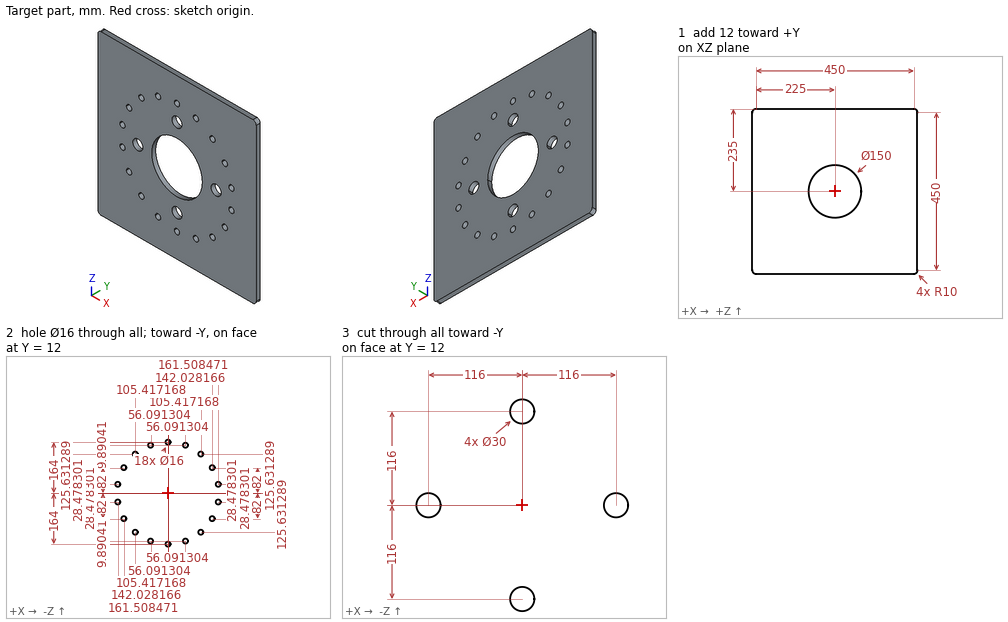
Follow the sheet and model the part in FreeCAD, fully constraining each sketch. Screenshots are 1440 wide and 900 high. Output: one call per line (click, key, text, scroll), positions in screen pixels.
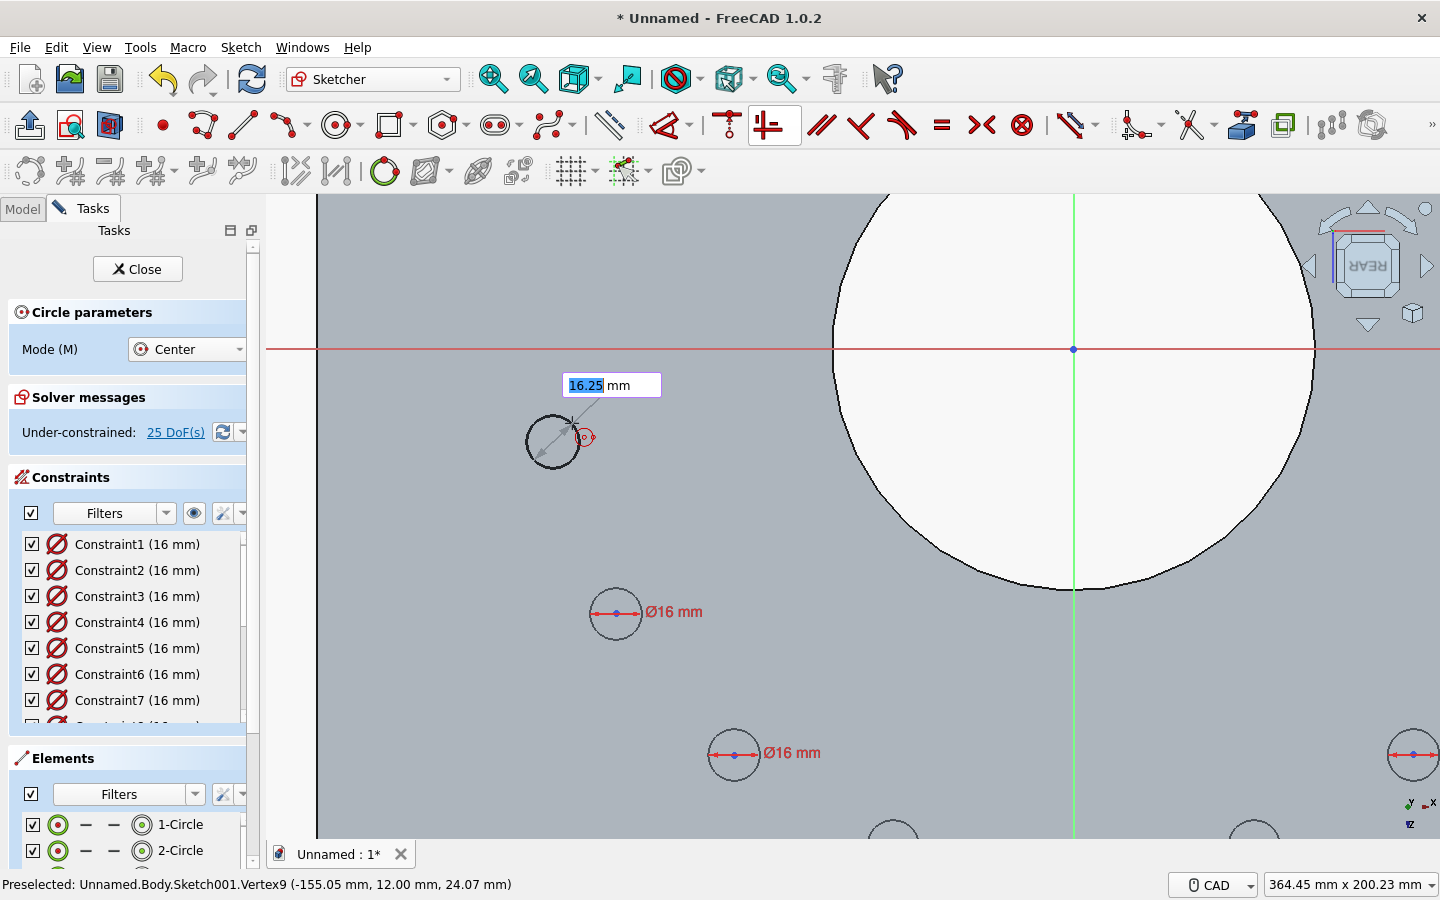
text(16)
key(Return)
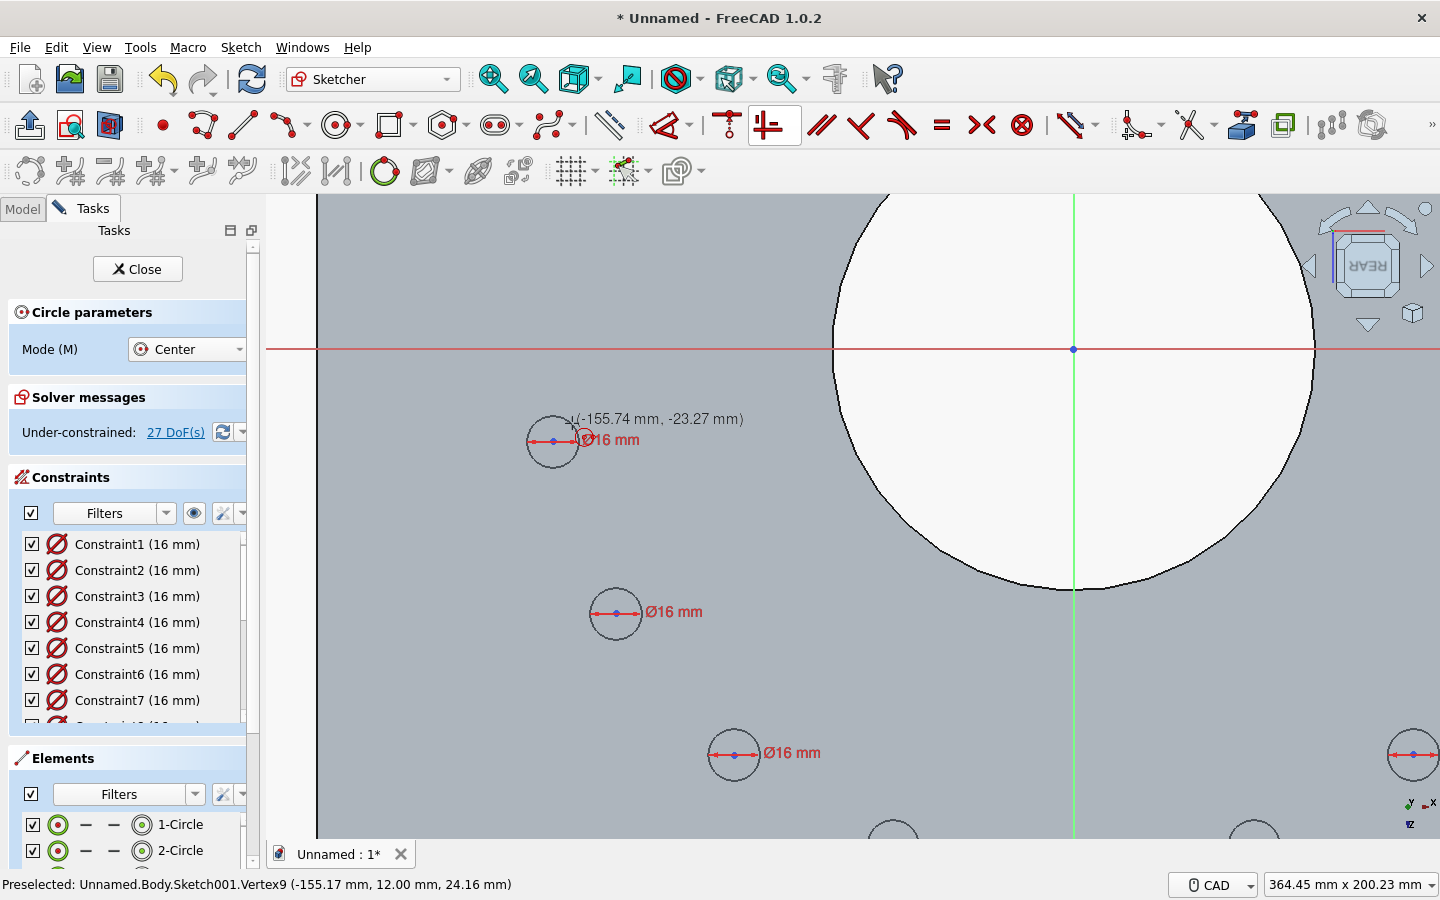
click(553, 257)
move(572, 239)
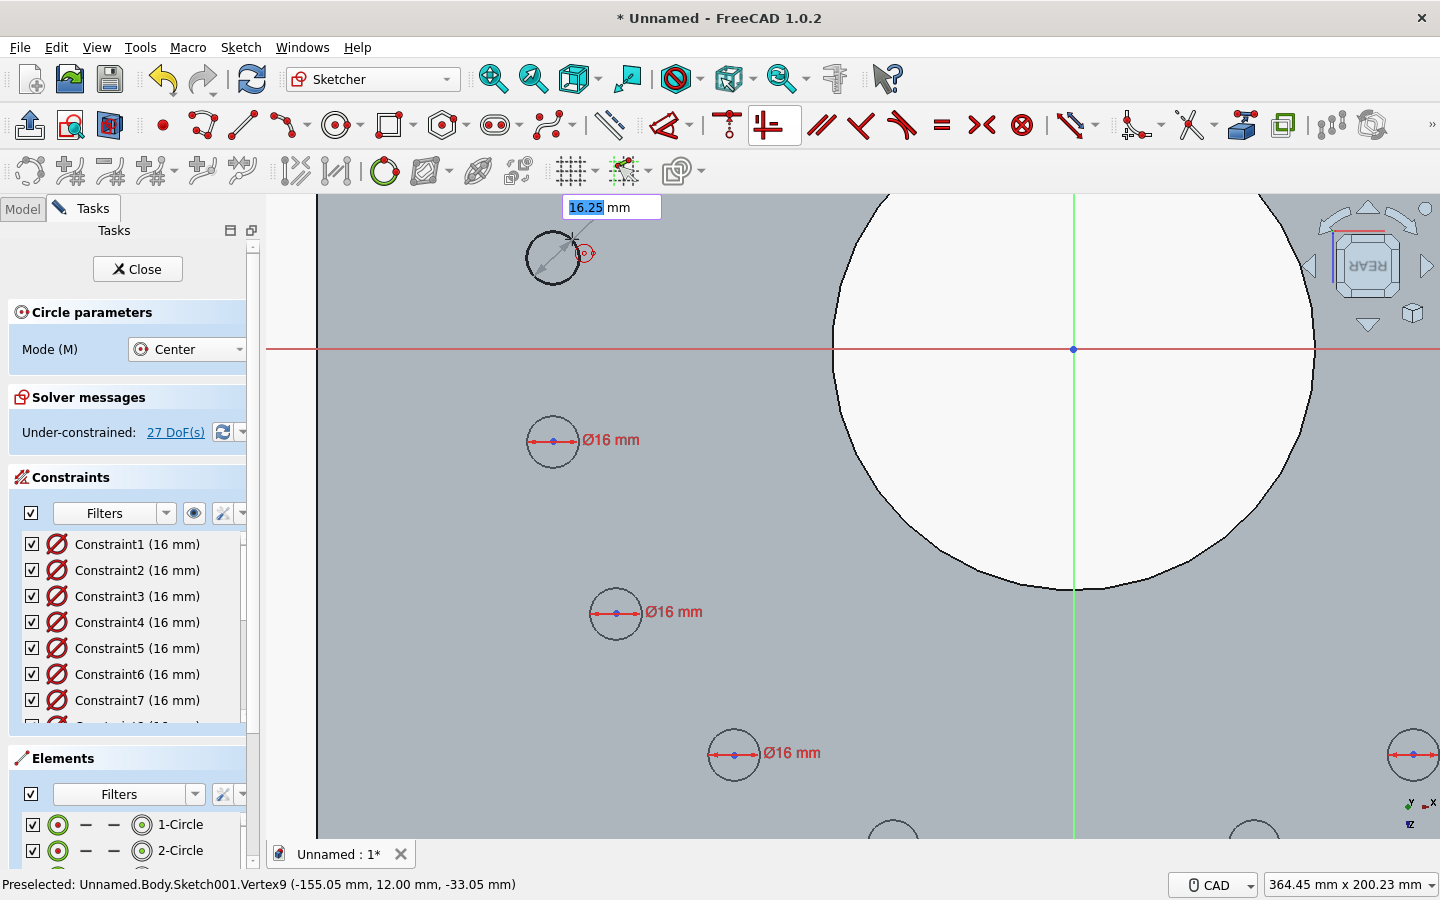
text(16)
key(Return)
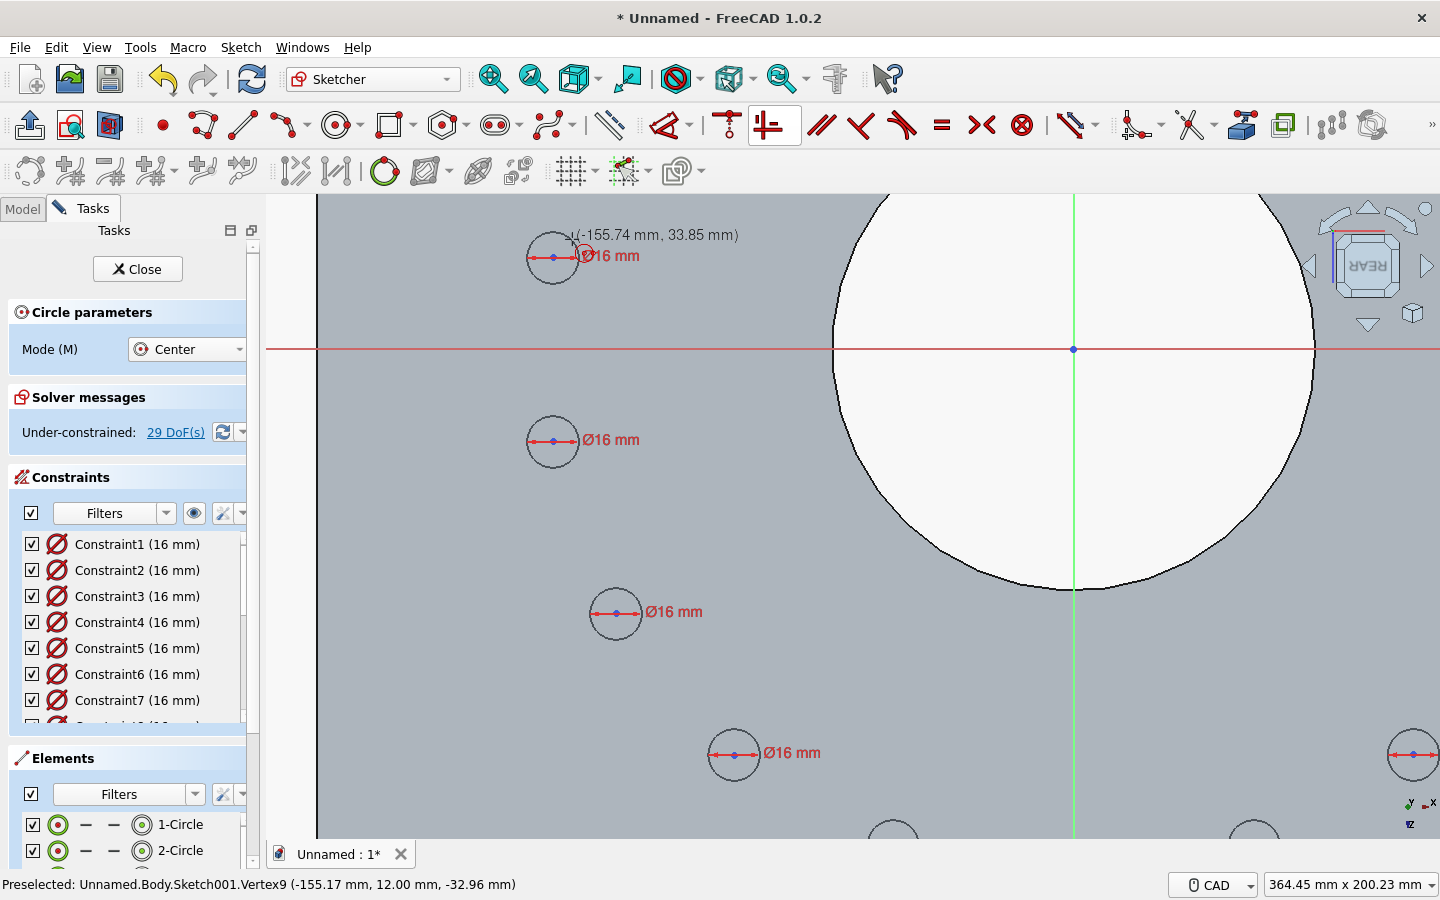
scroll(616, 614, down, 5)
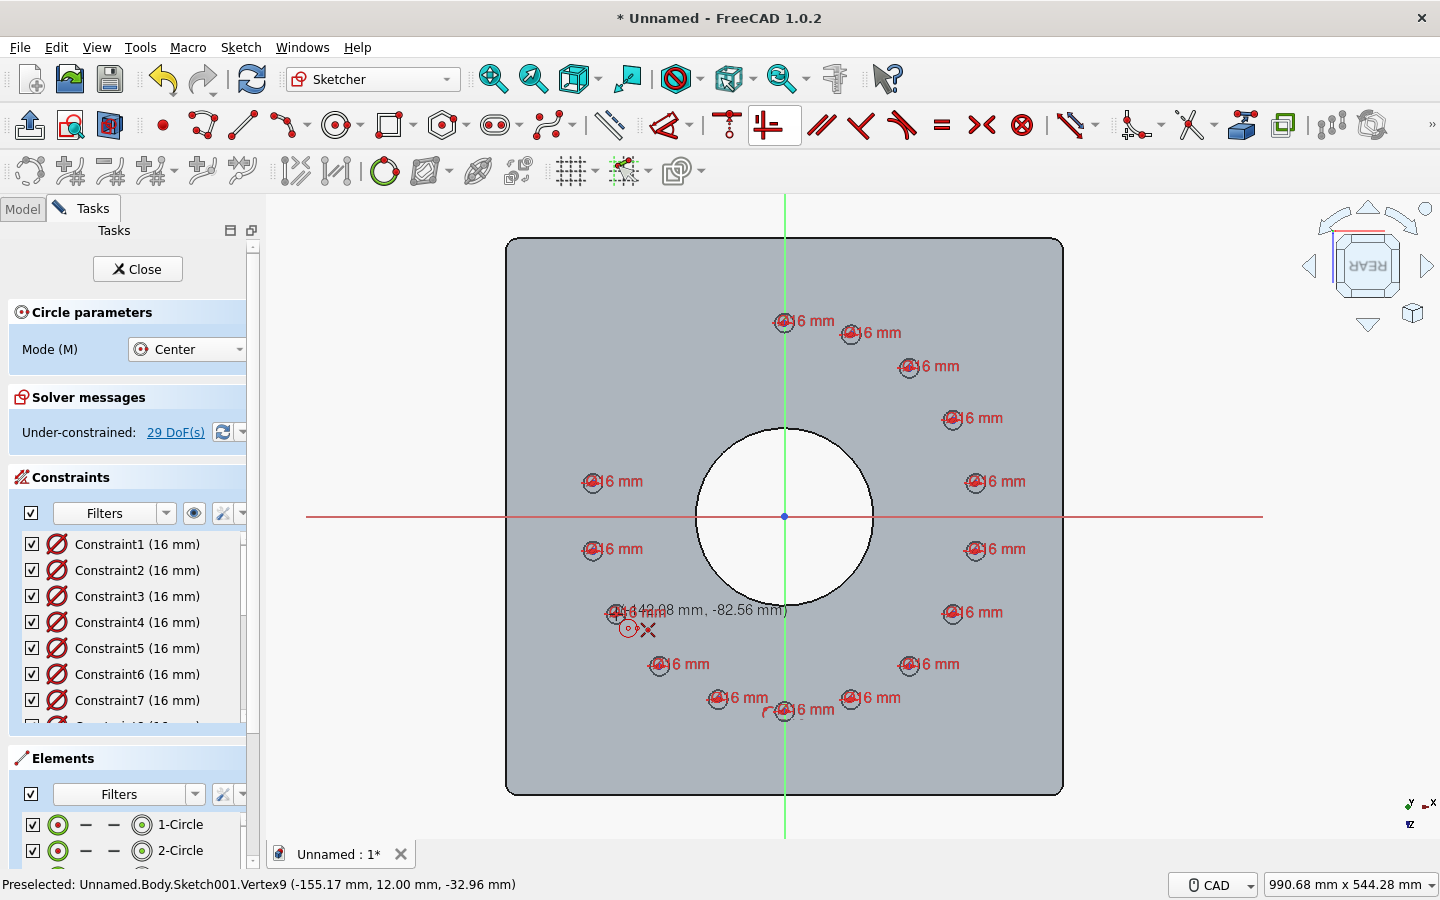
scroll(616, 420, up, 5)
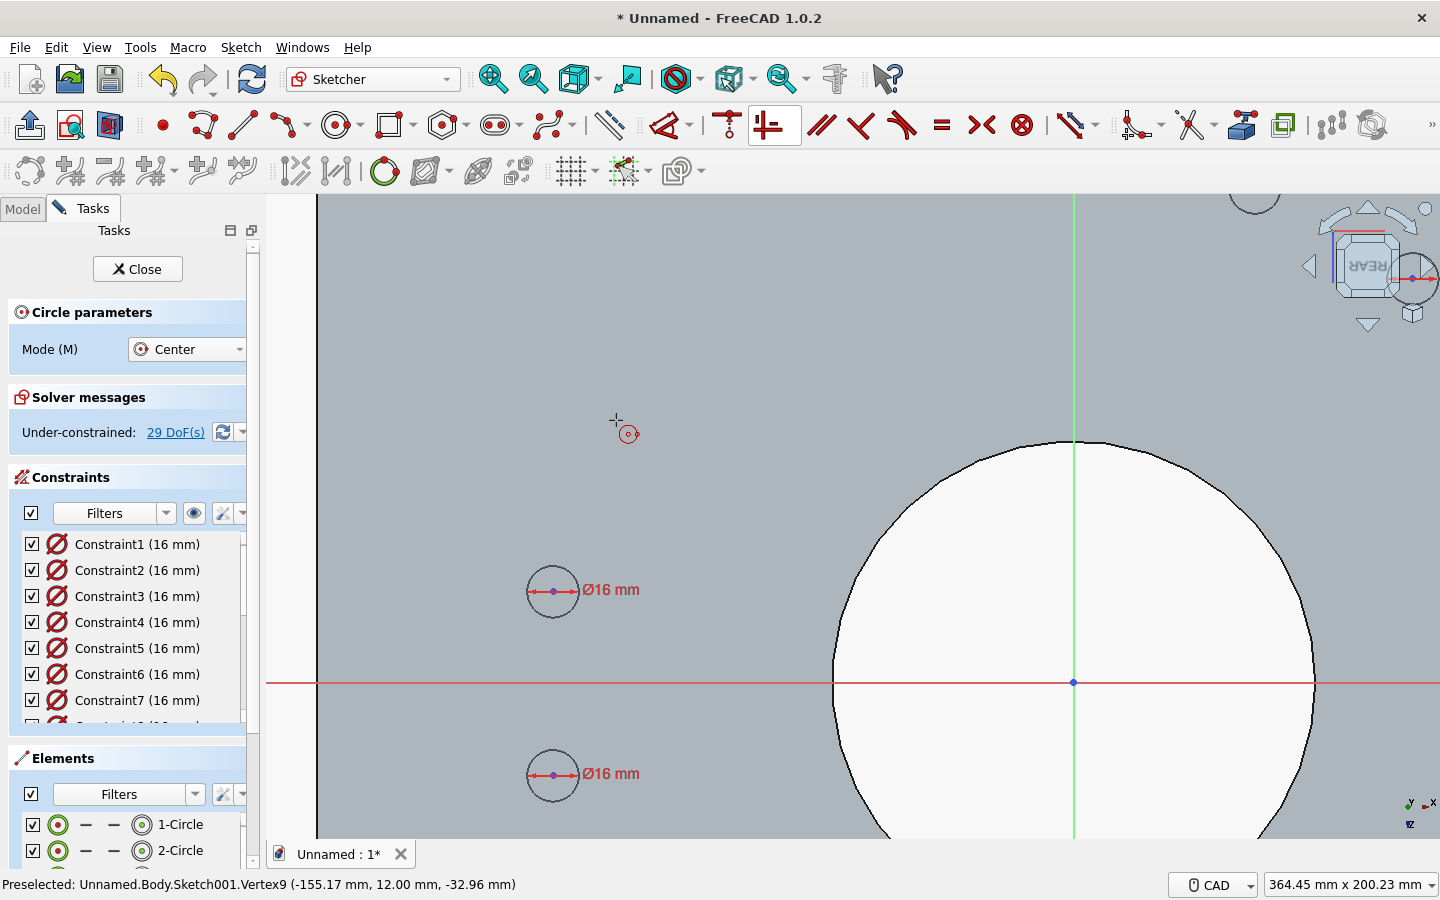
click(616, 419)
move(634, 401)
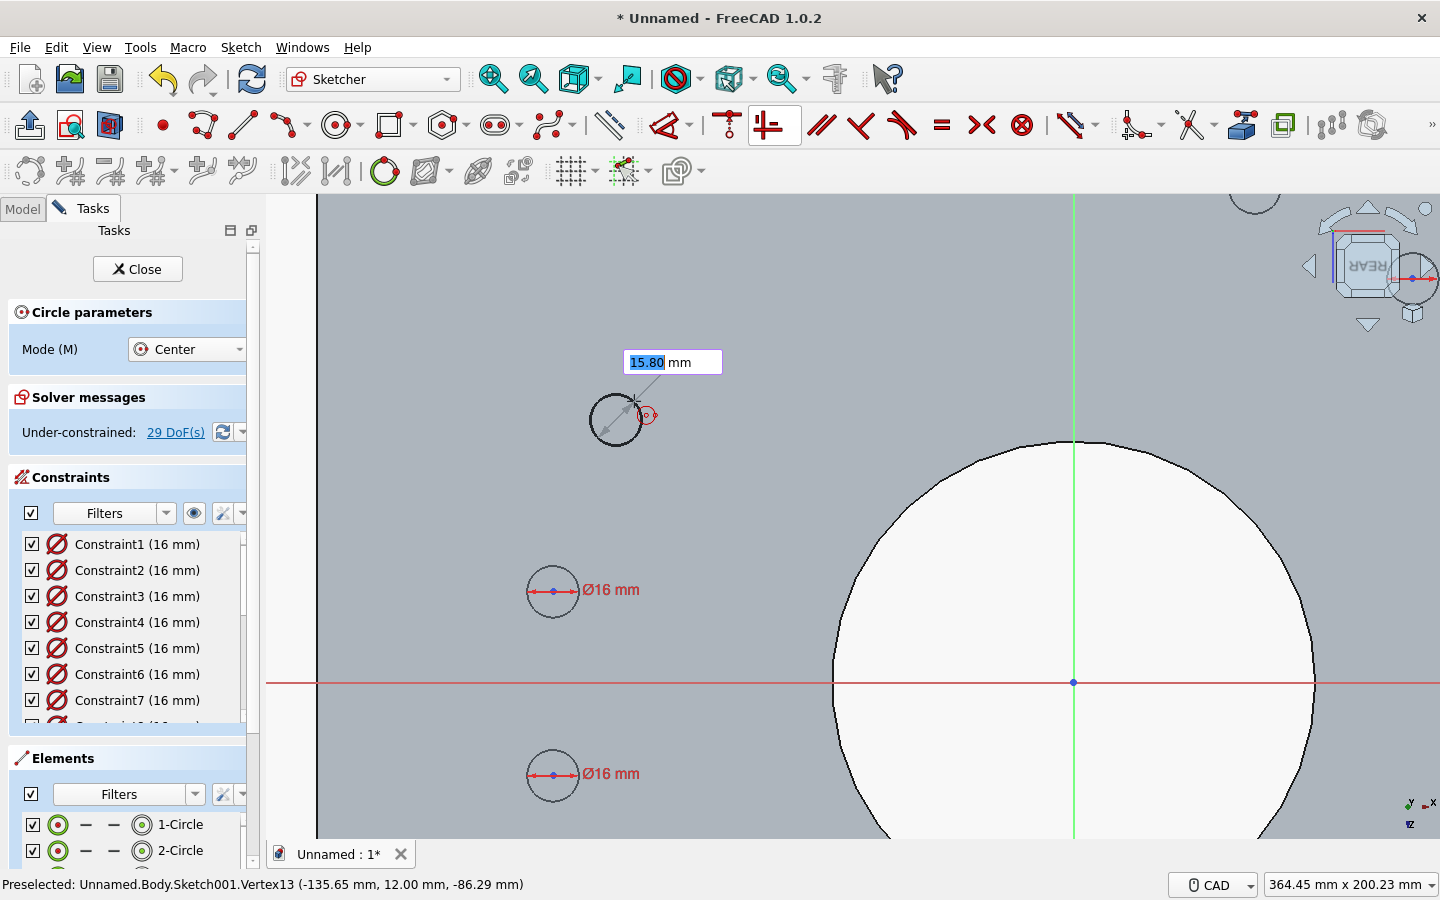
text(16)
key(Return)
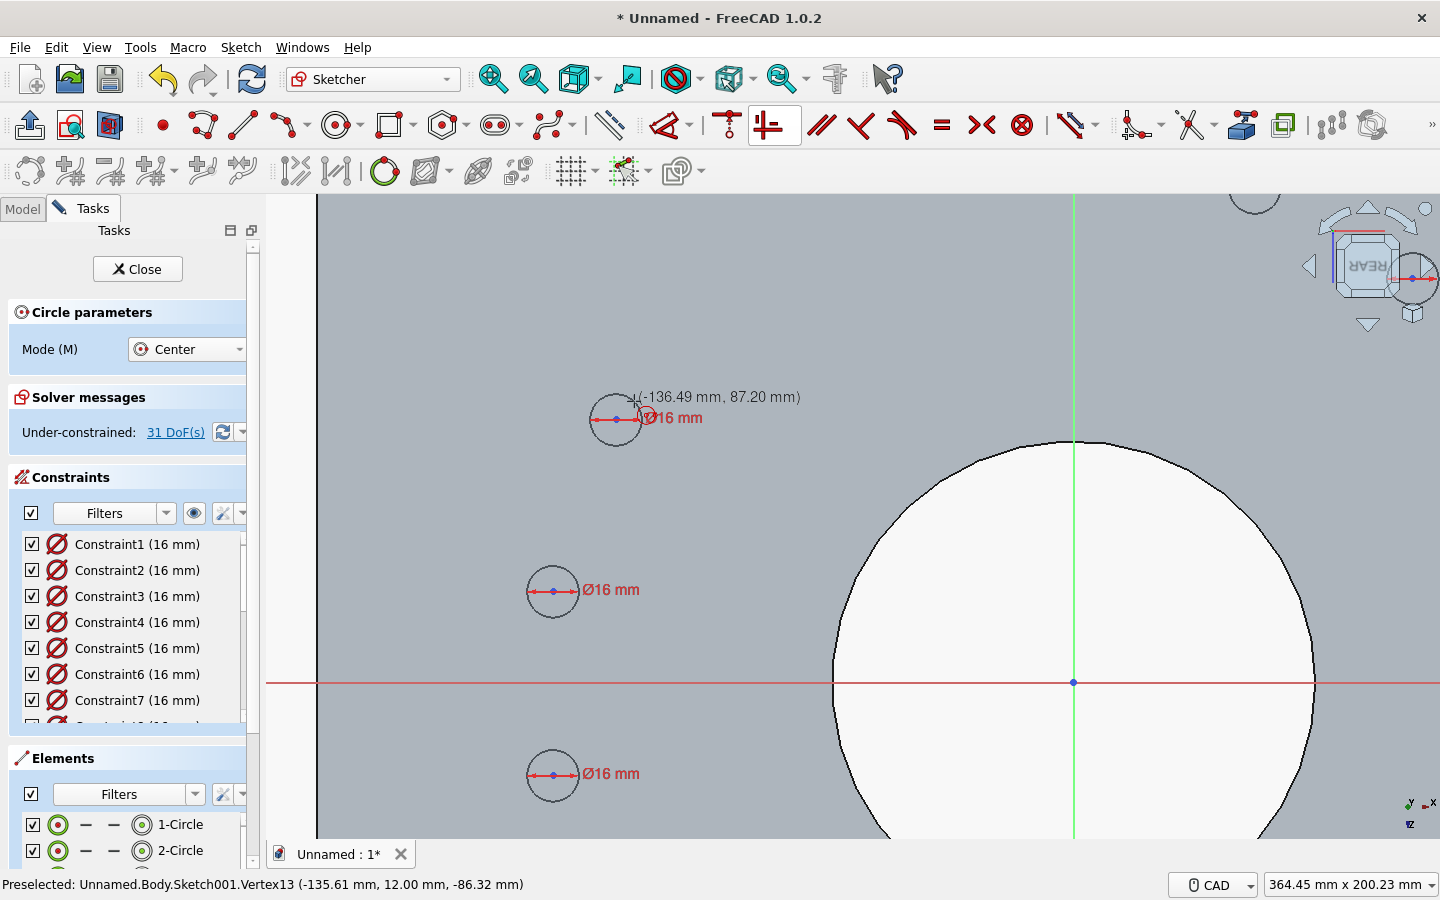
click(734, 278)
move(752, 260)